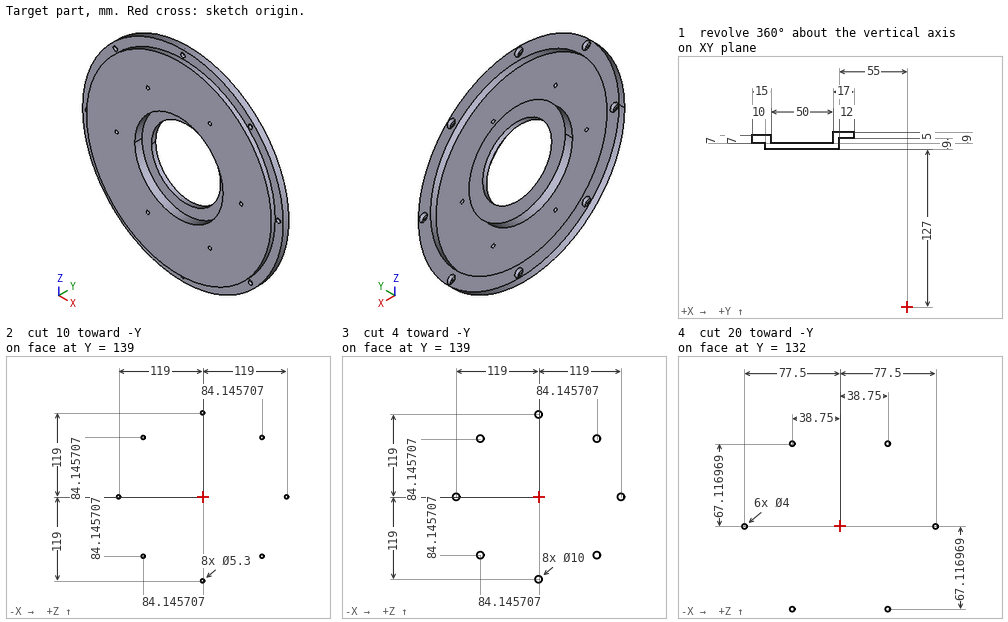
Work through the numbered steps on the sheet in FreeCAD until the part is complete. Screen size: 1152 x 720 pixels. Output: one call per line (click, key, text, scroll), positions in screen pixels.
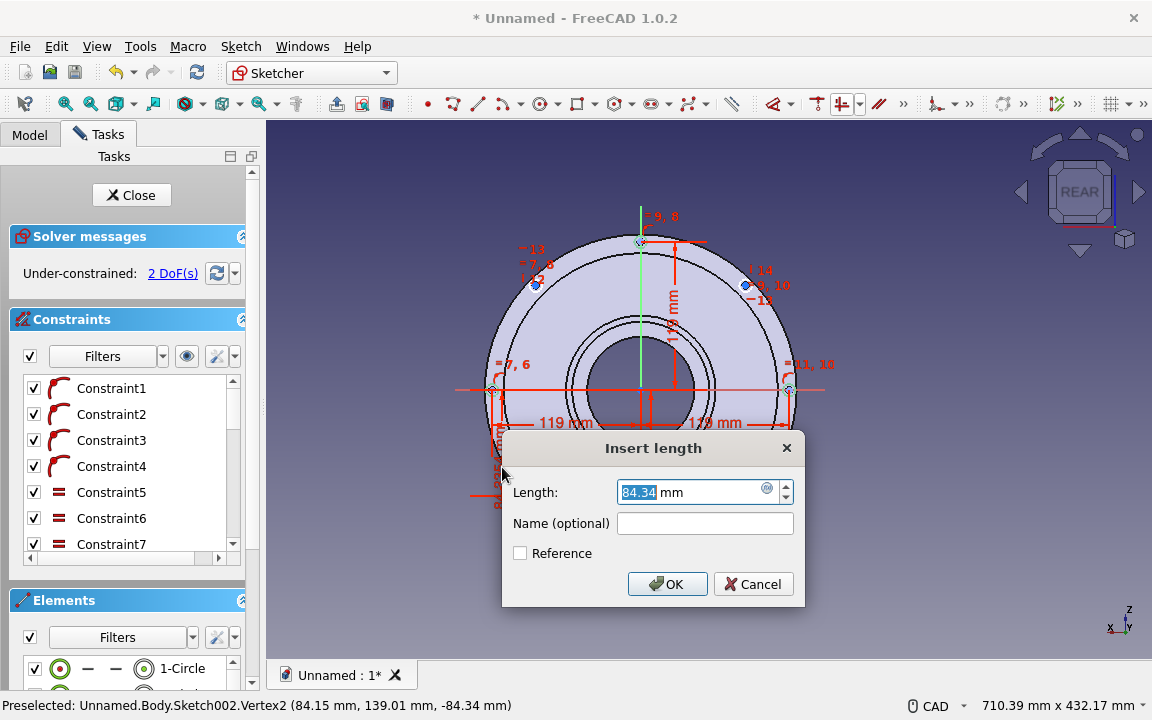
text(84.145707)
key(Return)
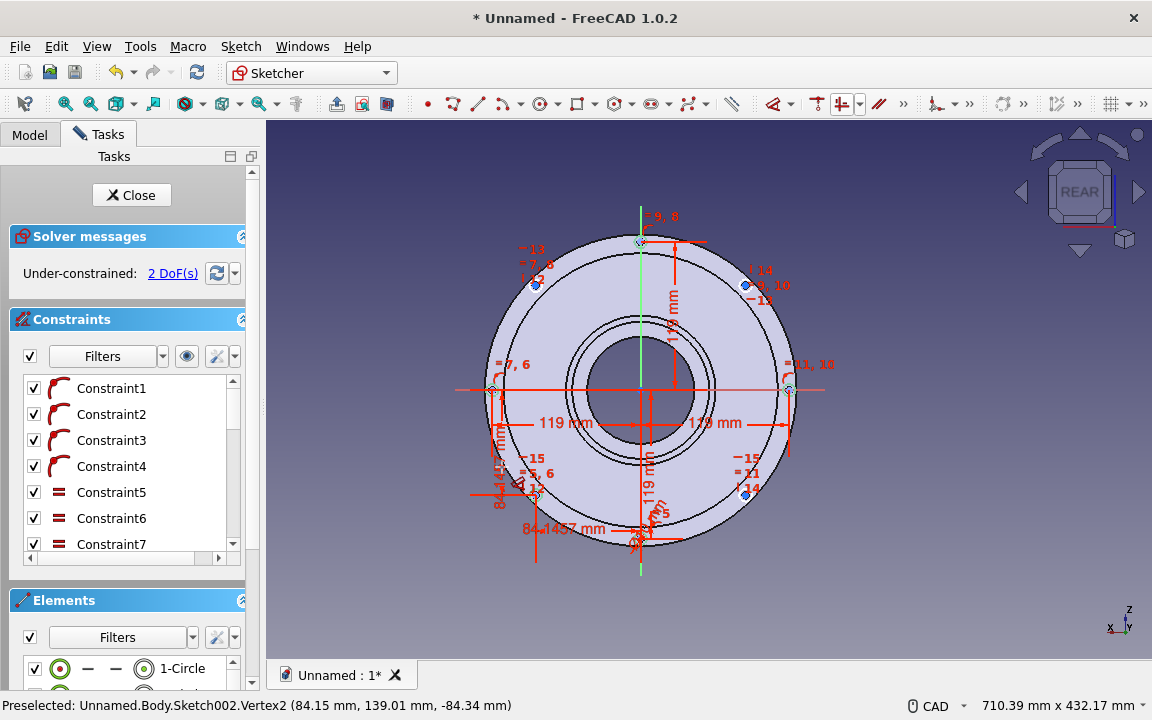
click(536, 286)
click(502, 338)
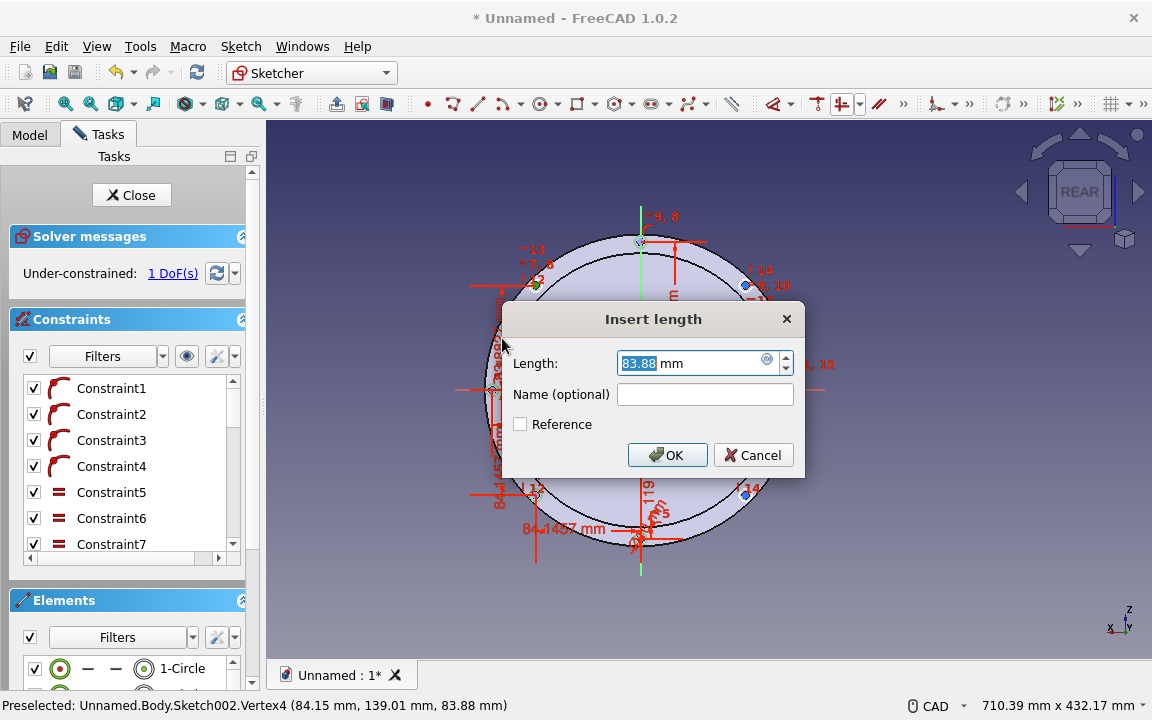
text(84.145707)
key(Return)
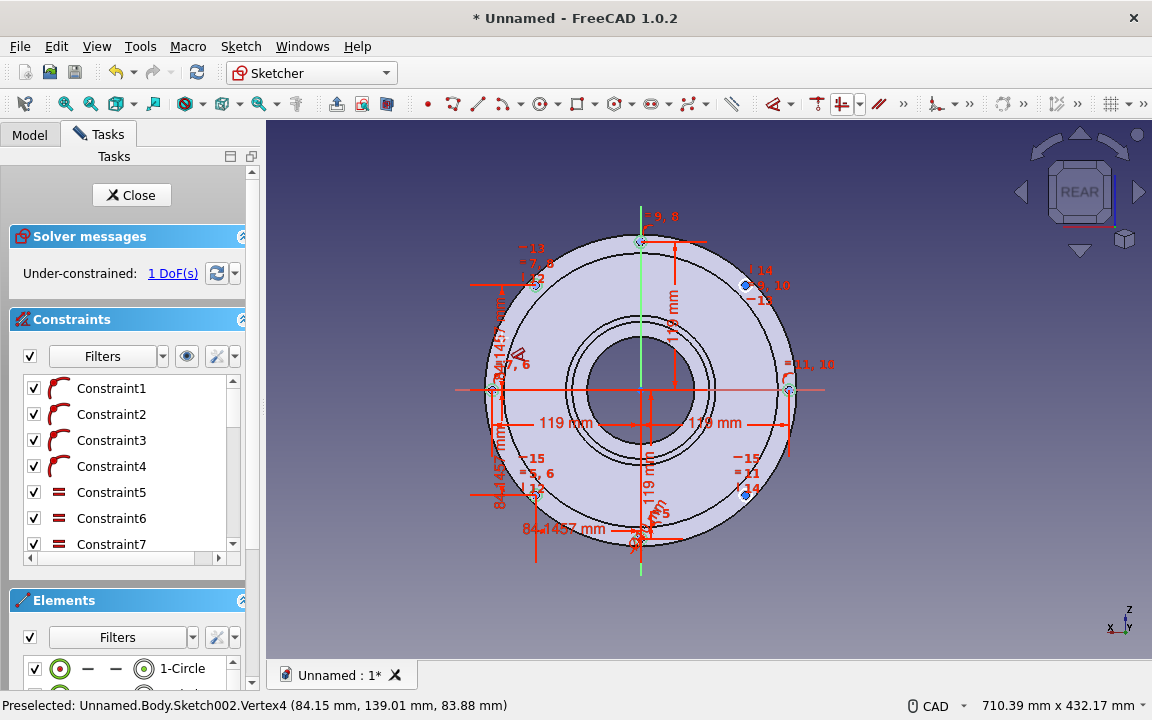
click(746, 285)
click(693, 251)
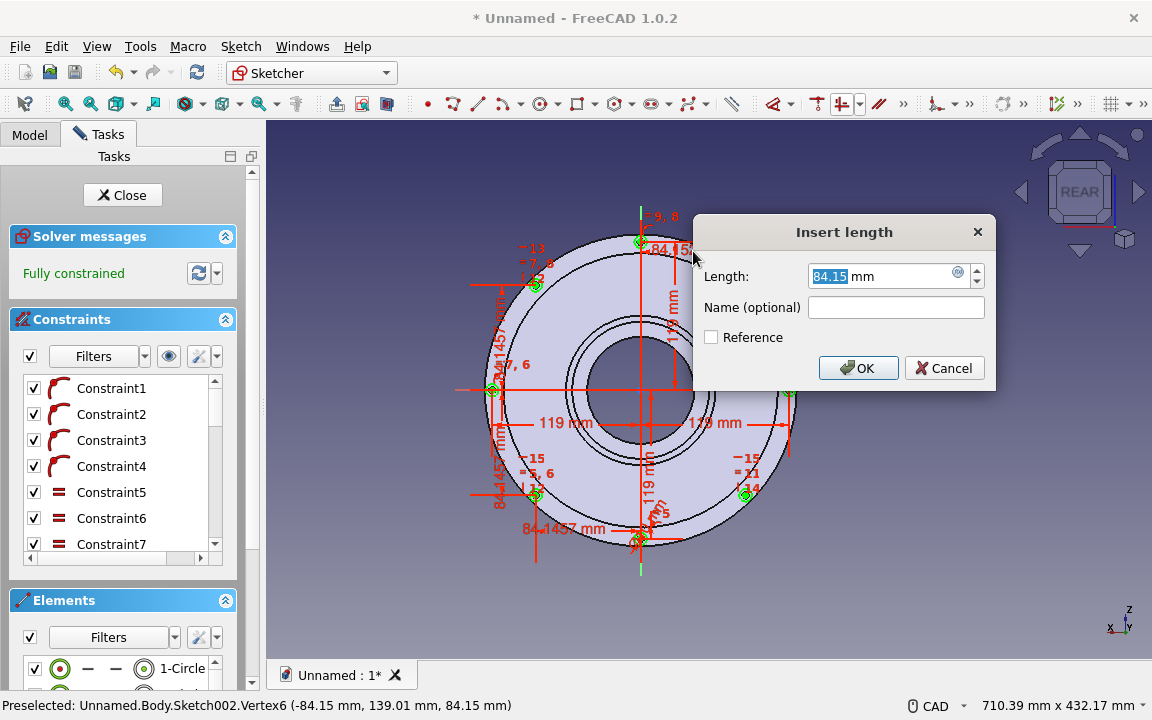
text(84.145707)
key(Return)
key(Escape)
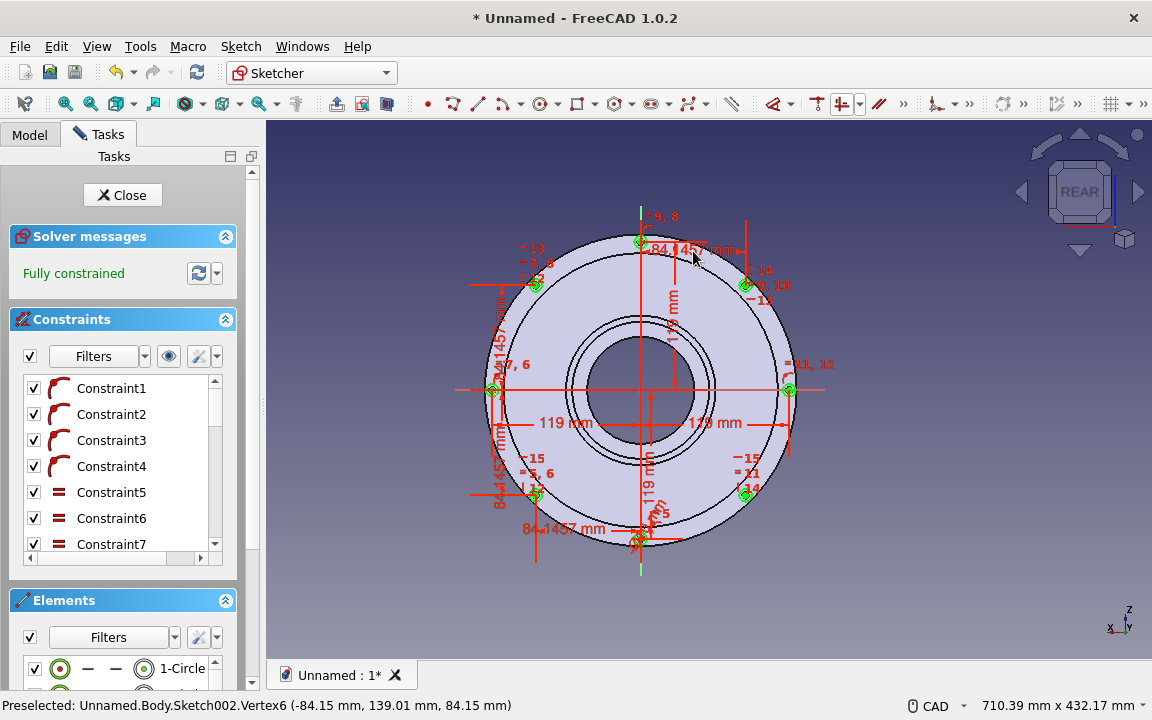
click(123, 195)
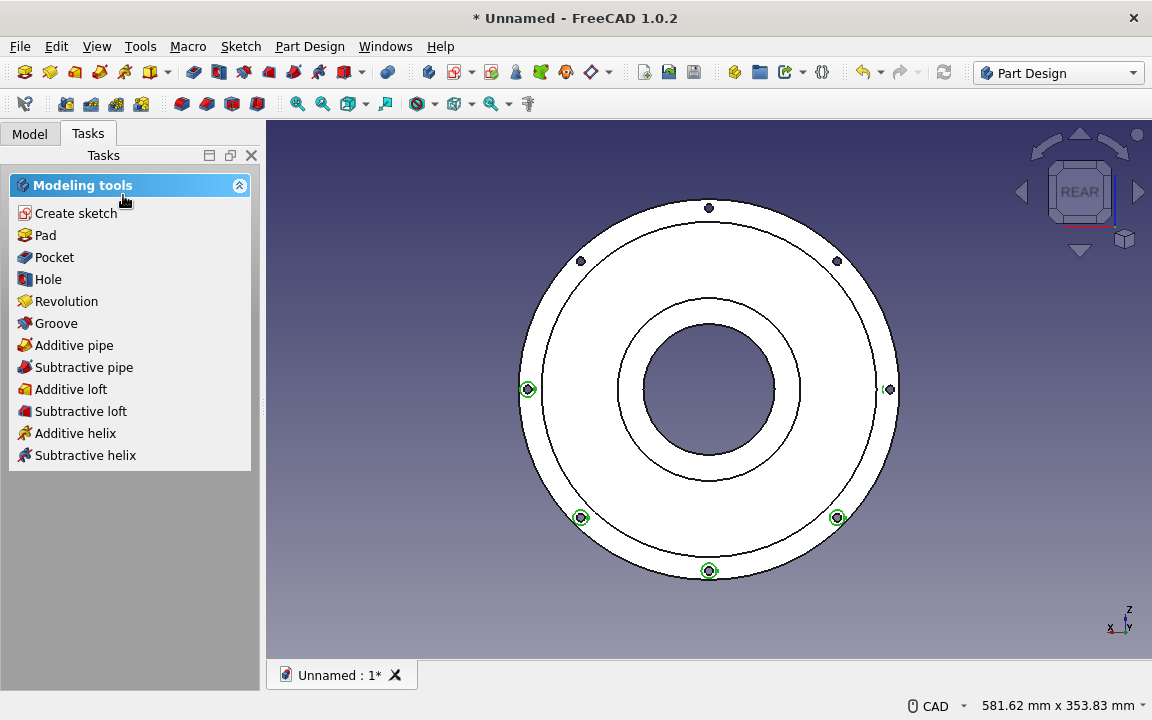
click(194, 72)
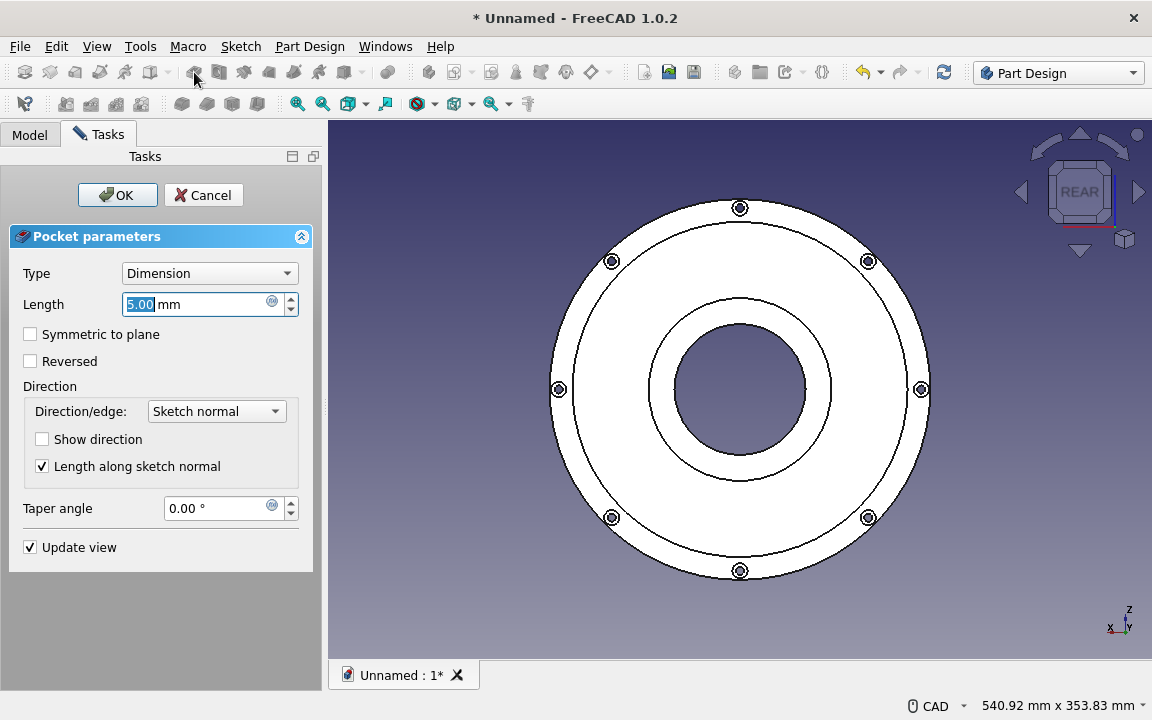
text(4)
key(Tab)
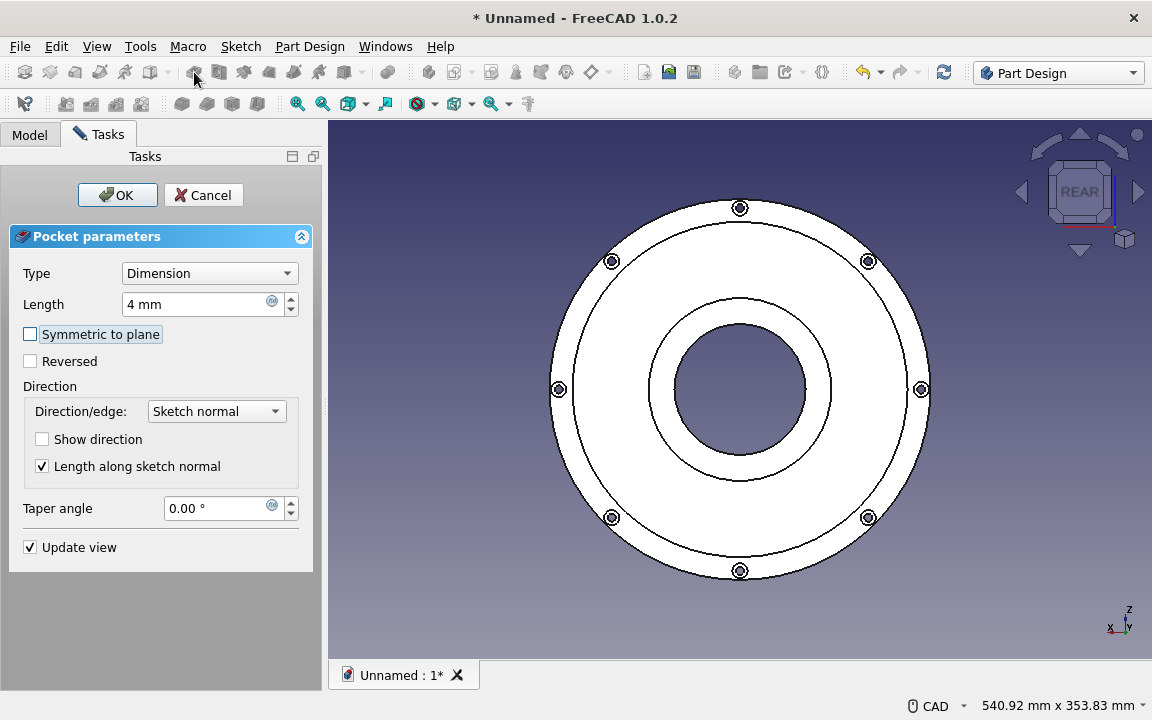
click(118, 195)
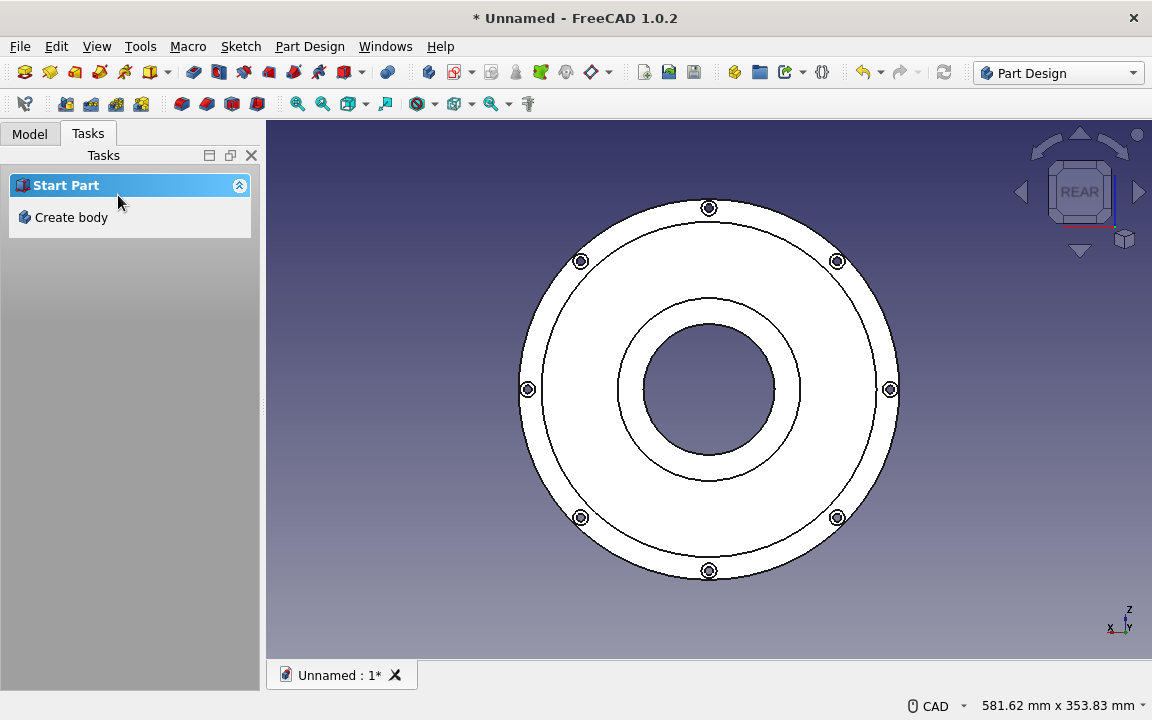
click(613, 484)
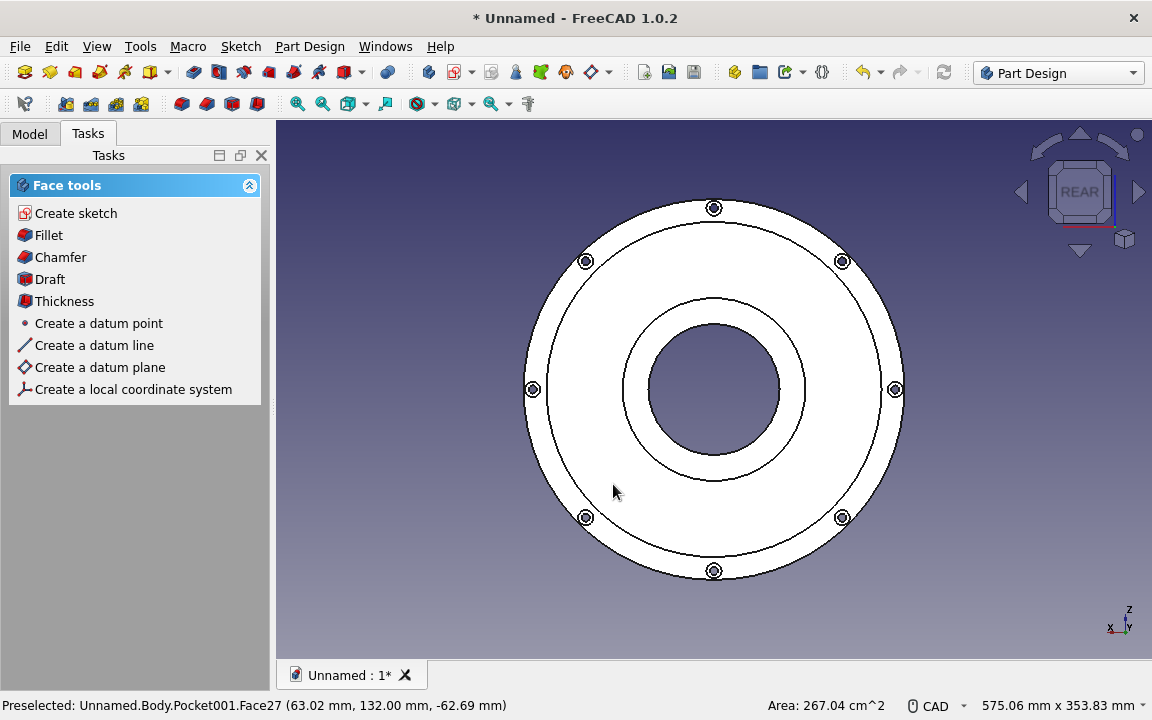
click(454, 72)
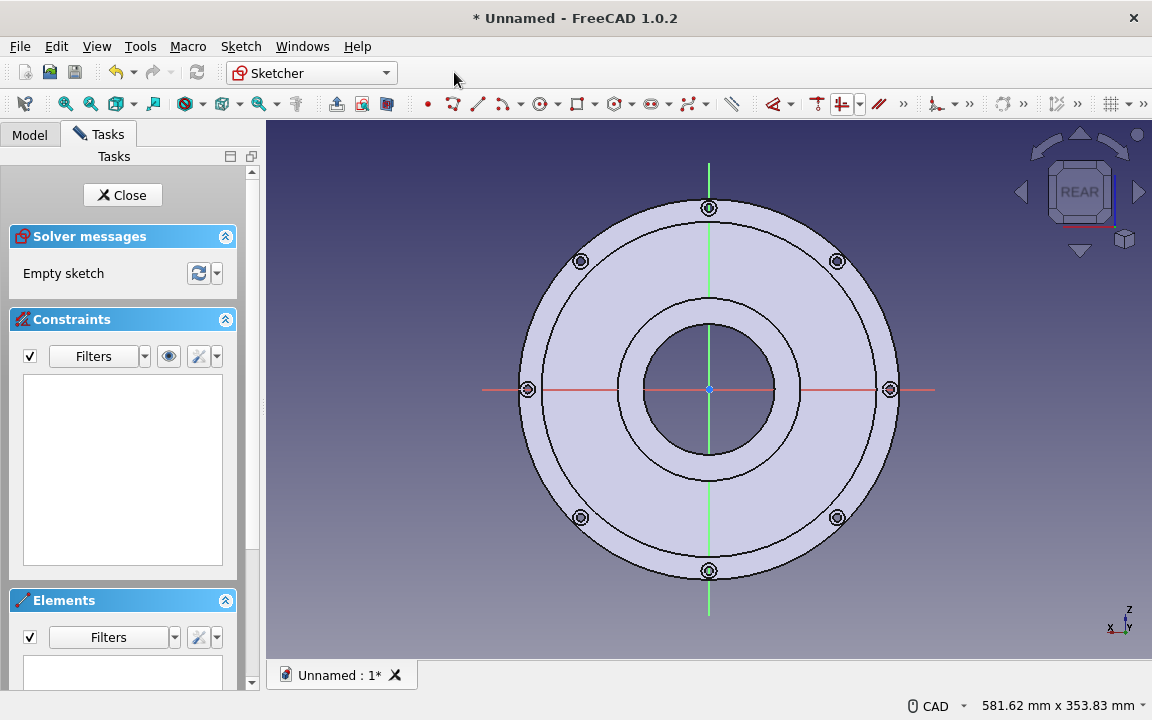
scroll(848, 390, up, 2)